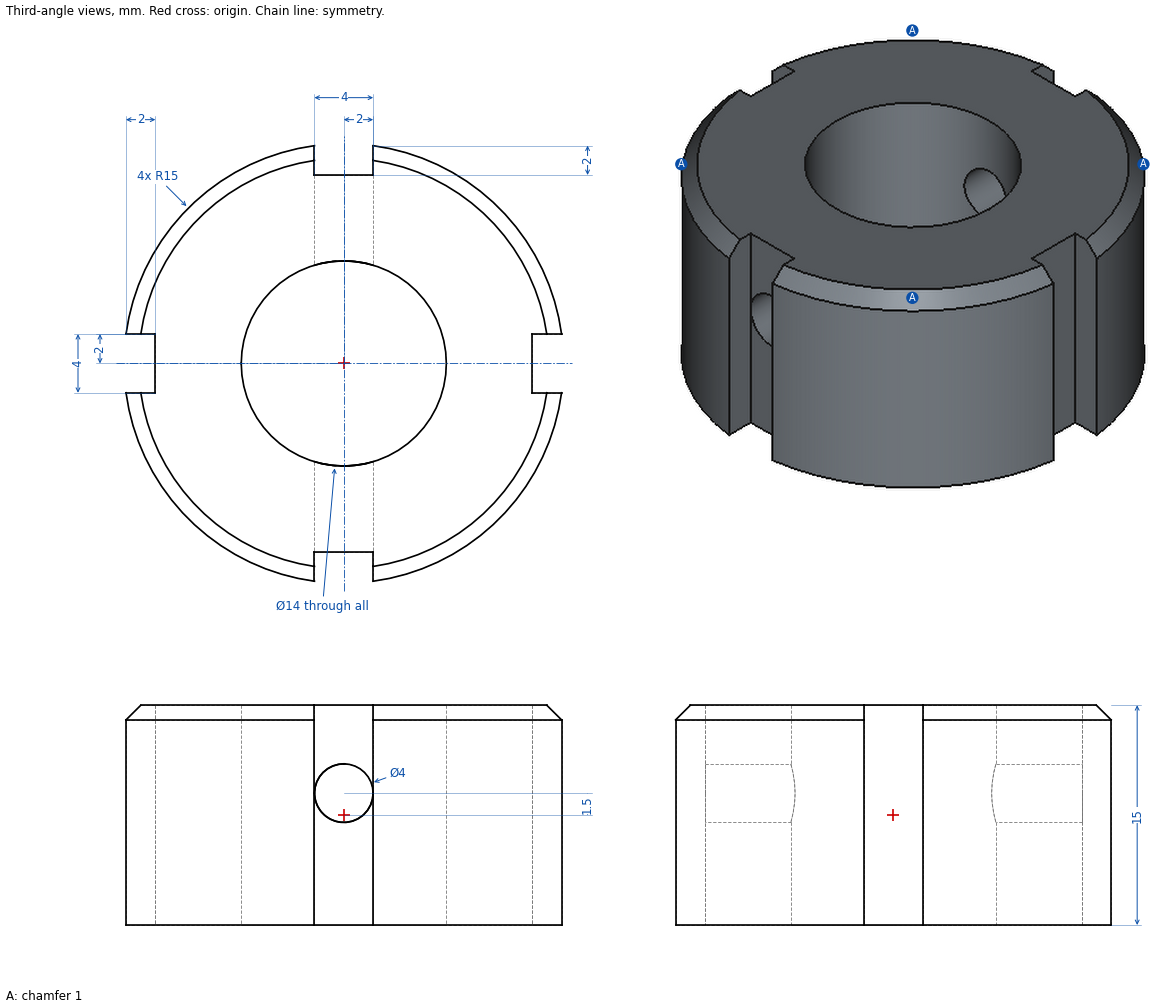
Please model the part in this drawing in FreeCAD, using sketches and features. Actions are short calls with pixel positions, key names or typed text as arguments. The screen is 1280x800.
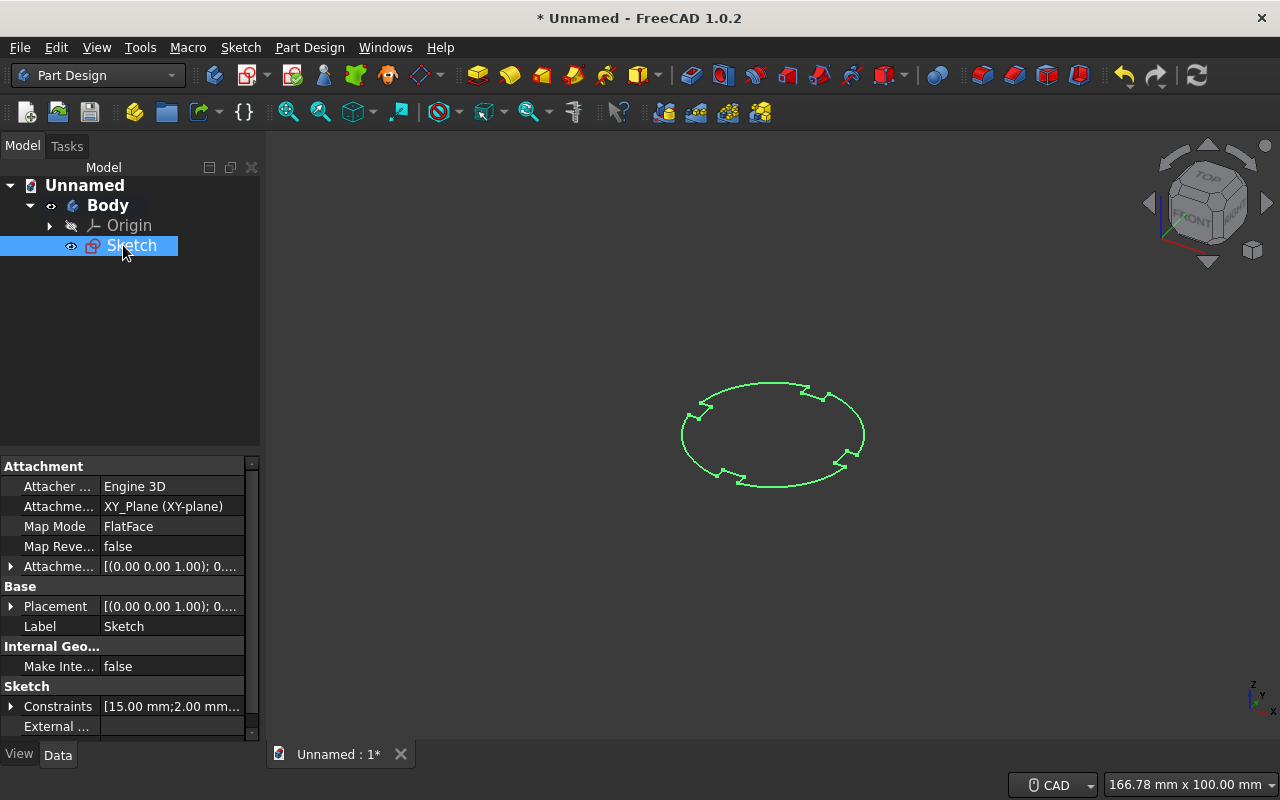
click(478, 76)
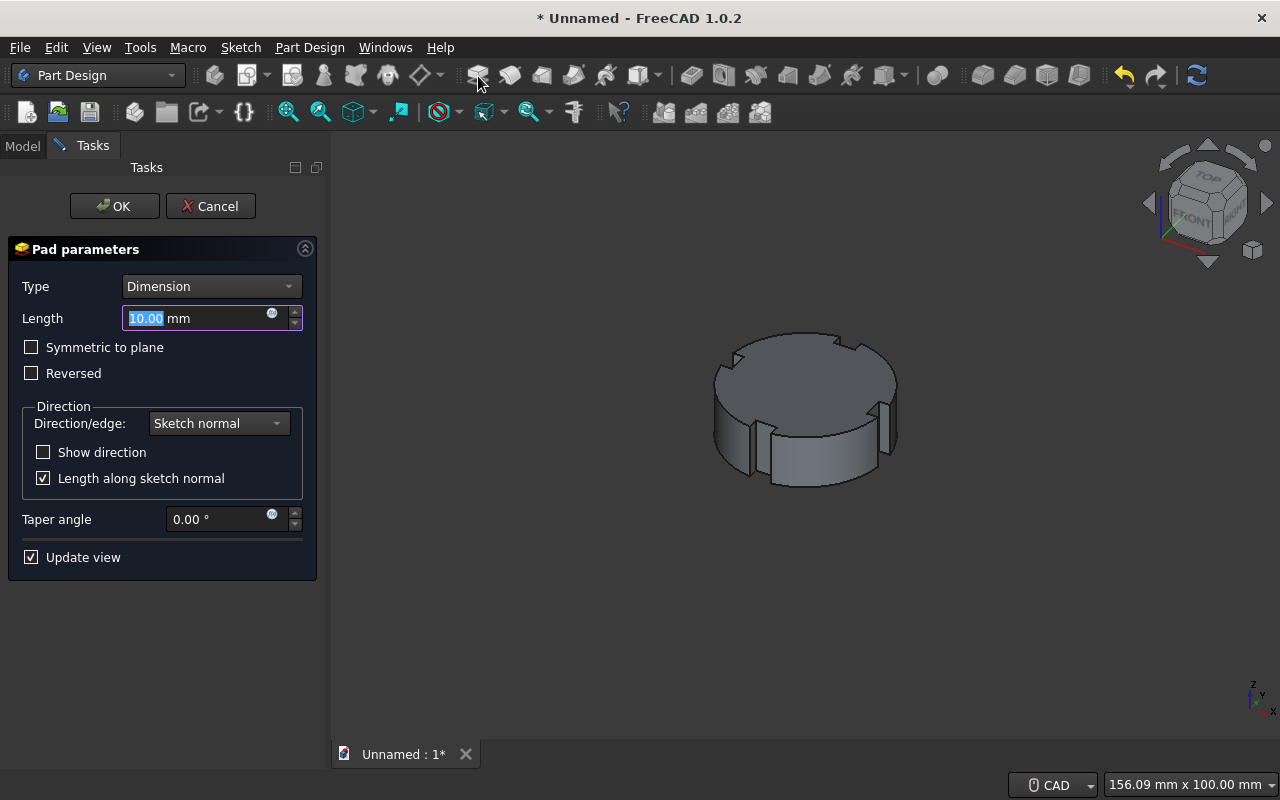
text(15)
key(Tab)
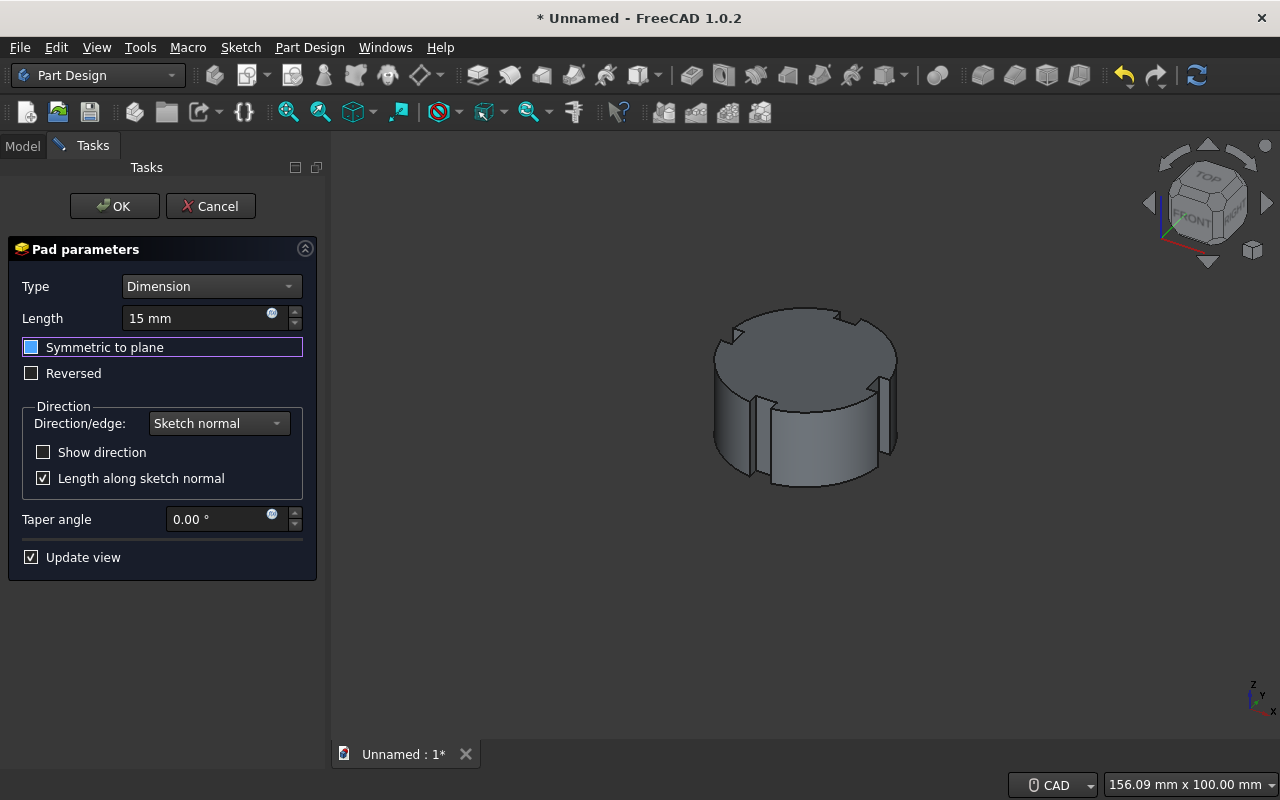
click(30, 347)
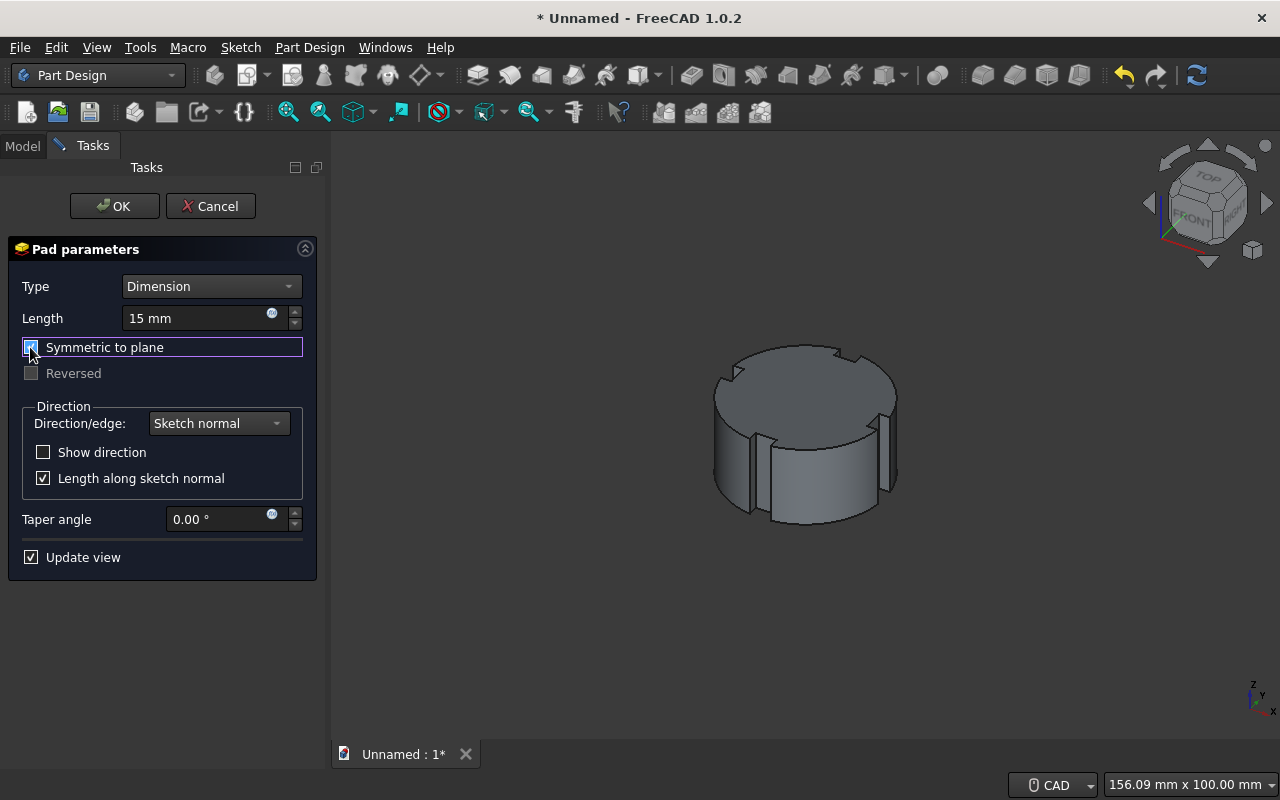
click(115, 206)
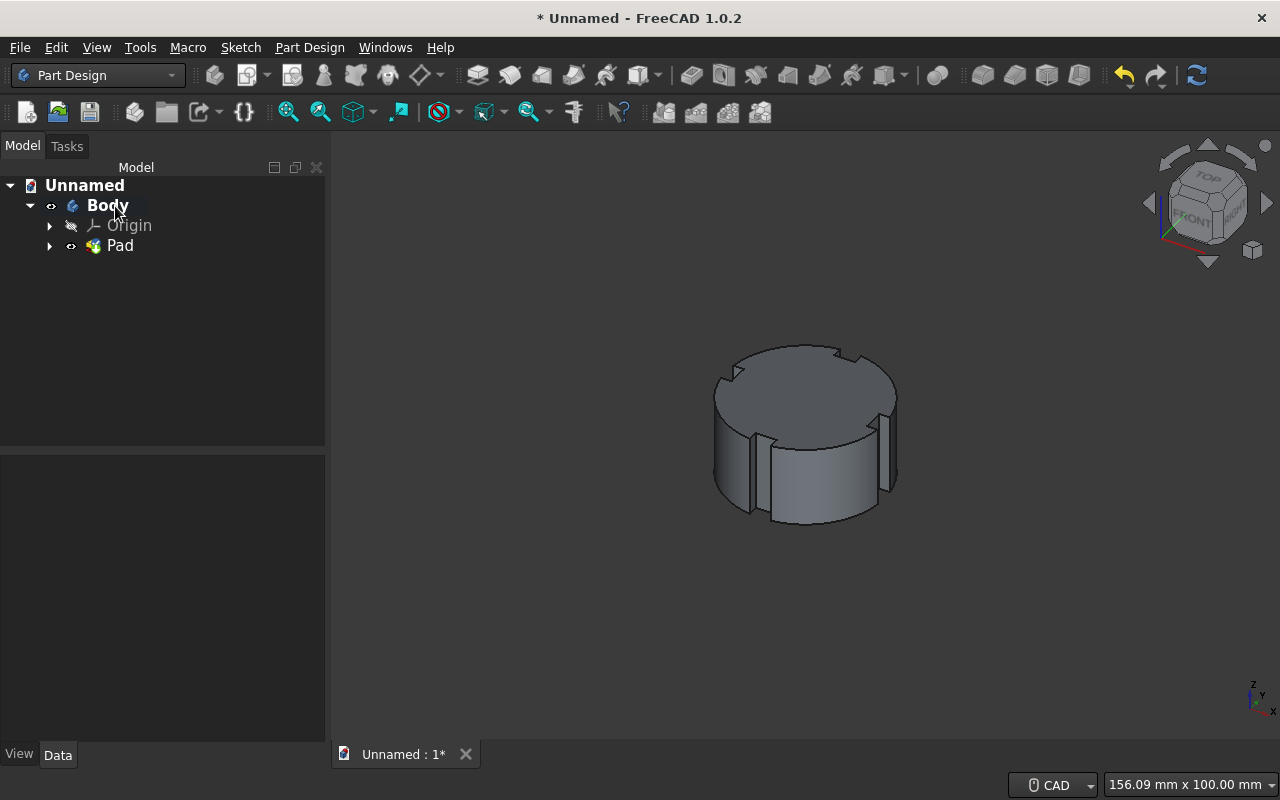
key(v)
key(f)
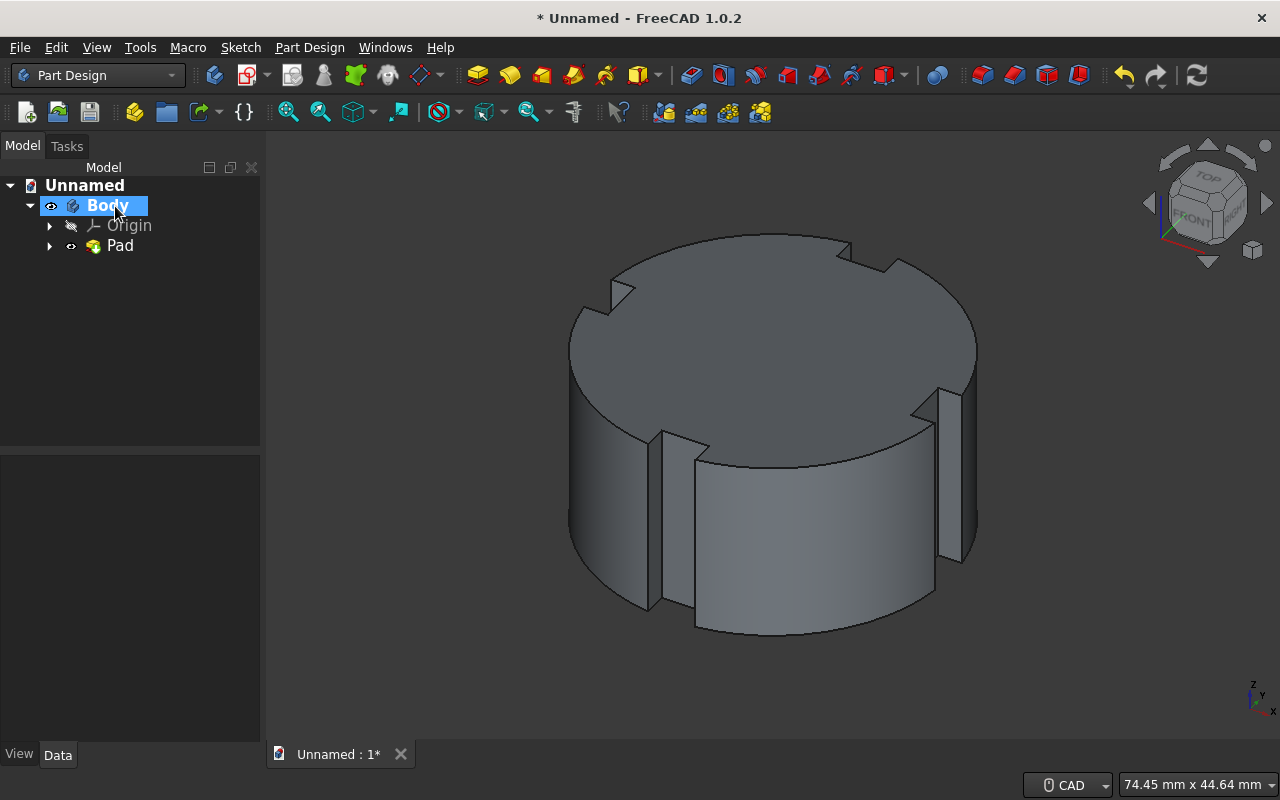
click(773, 350)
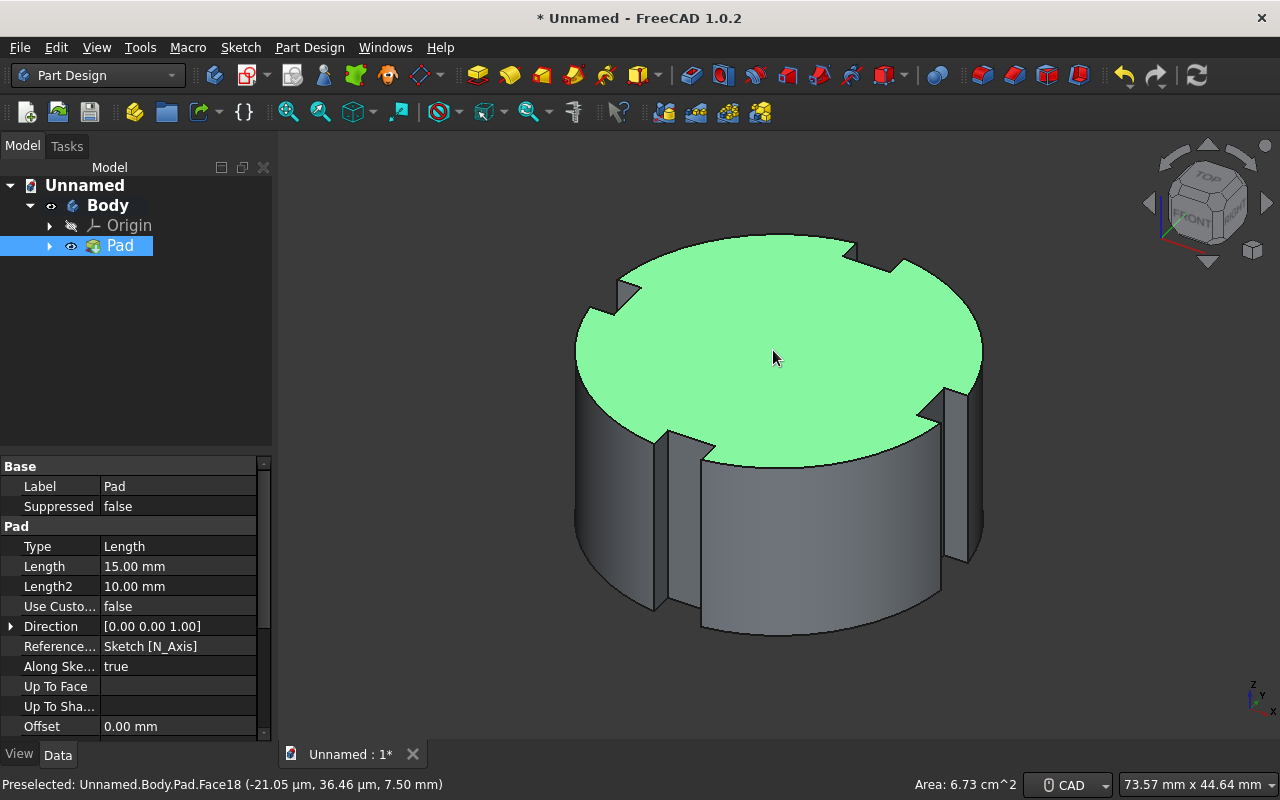
click(248, 76)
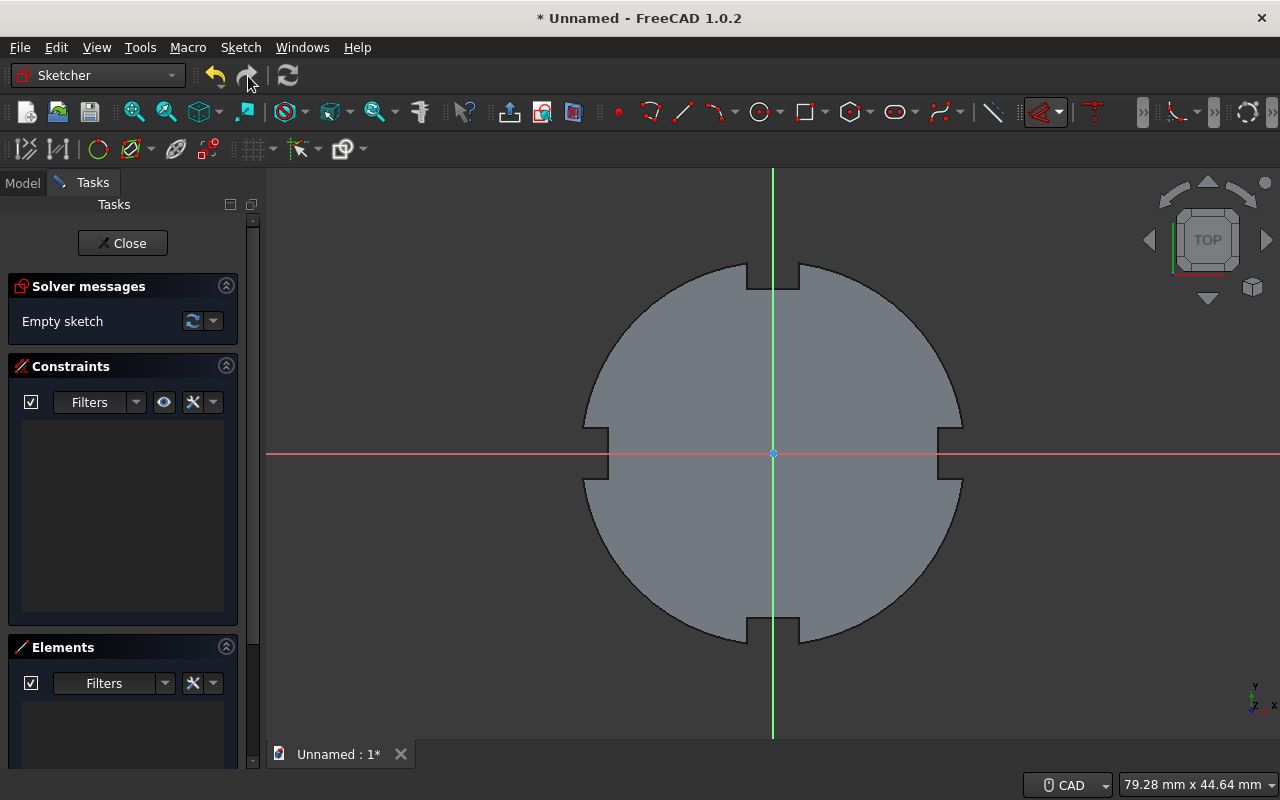
scroll(829, 454, up, 4)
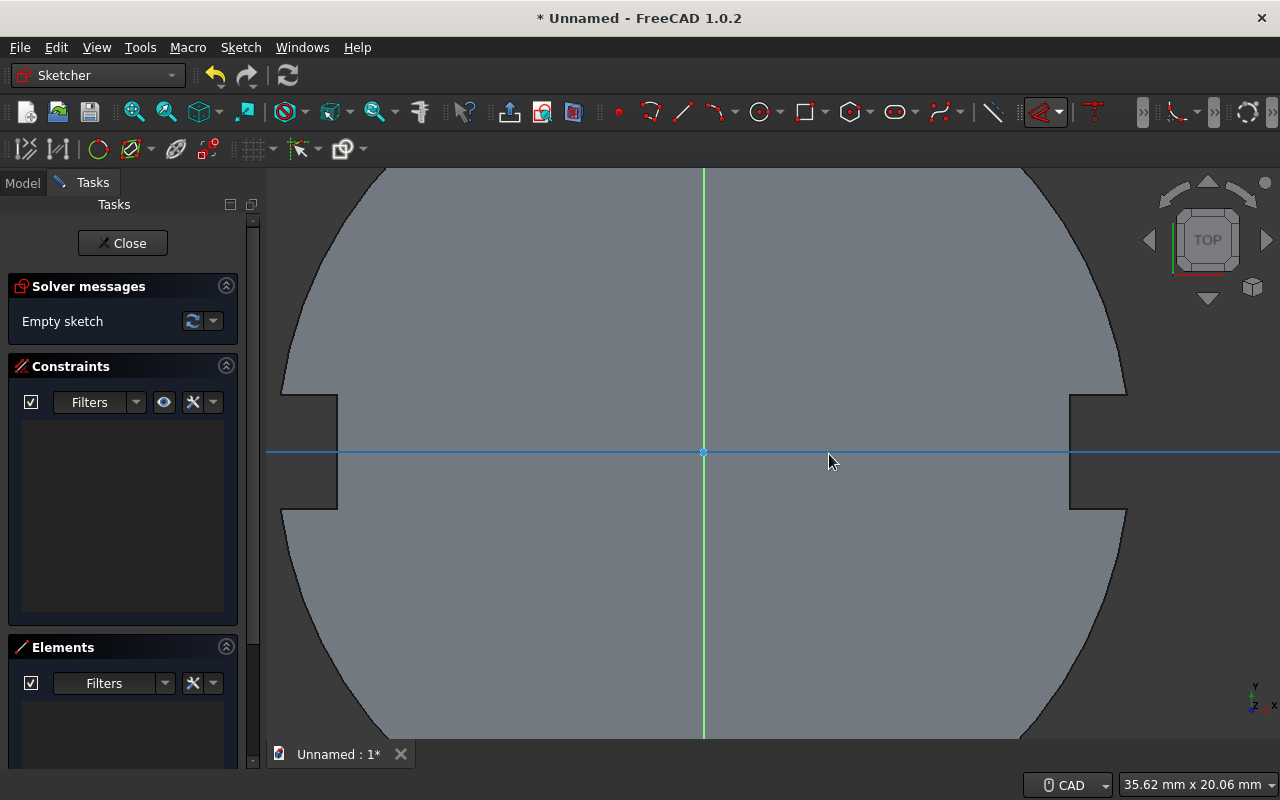
click(760, 112)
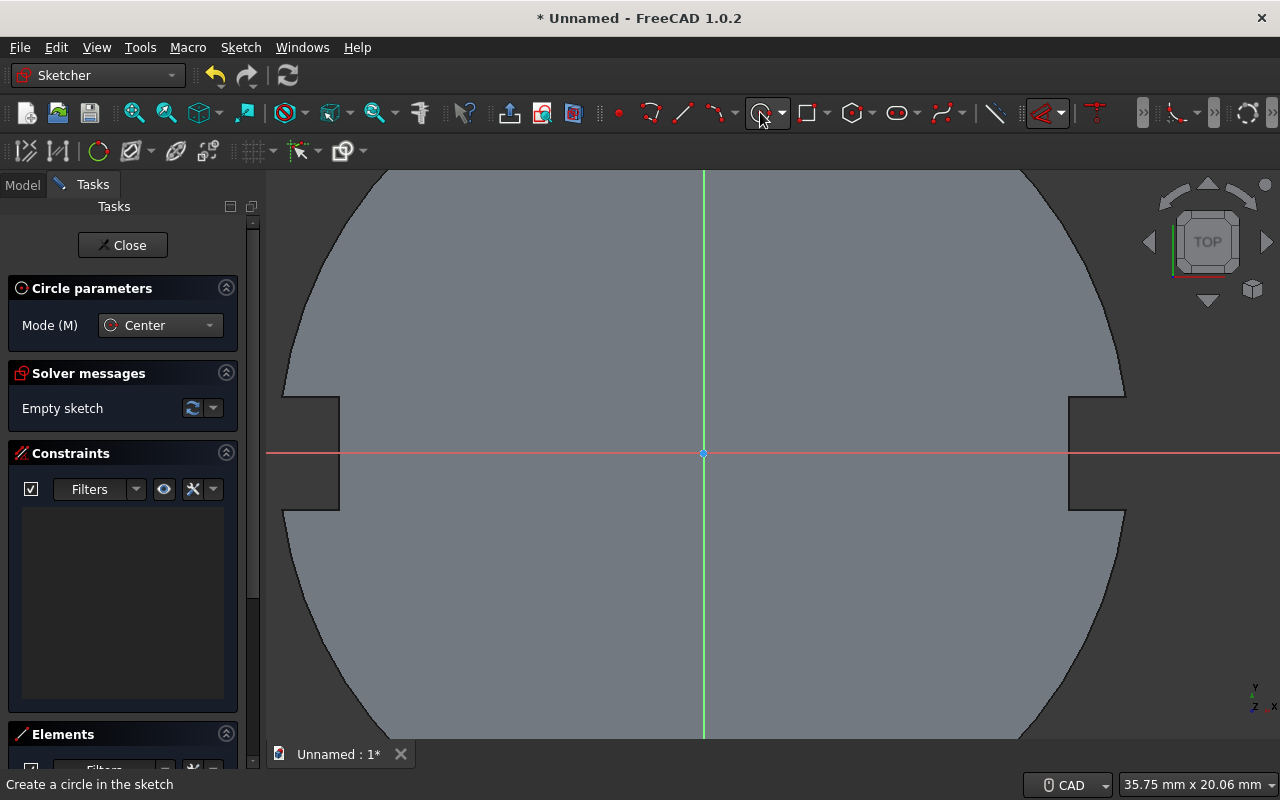
click(704, 453)
move(844, 313)